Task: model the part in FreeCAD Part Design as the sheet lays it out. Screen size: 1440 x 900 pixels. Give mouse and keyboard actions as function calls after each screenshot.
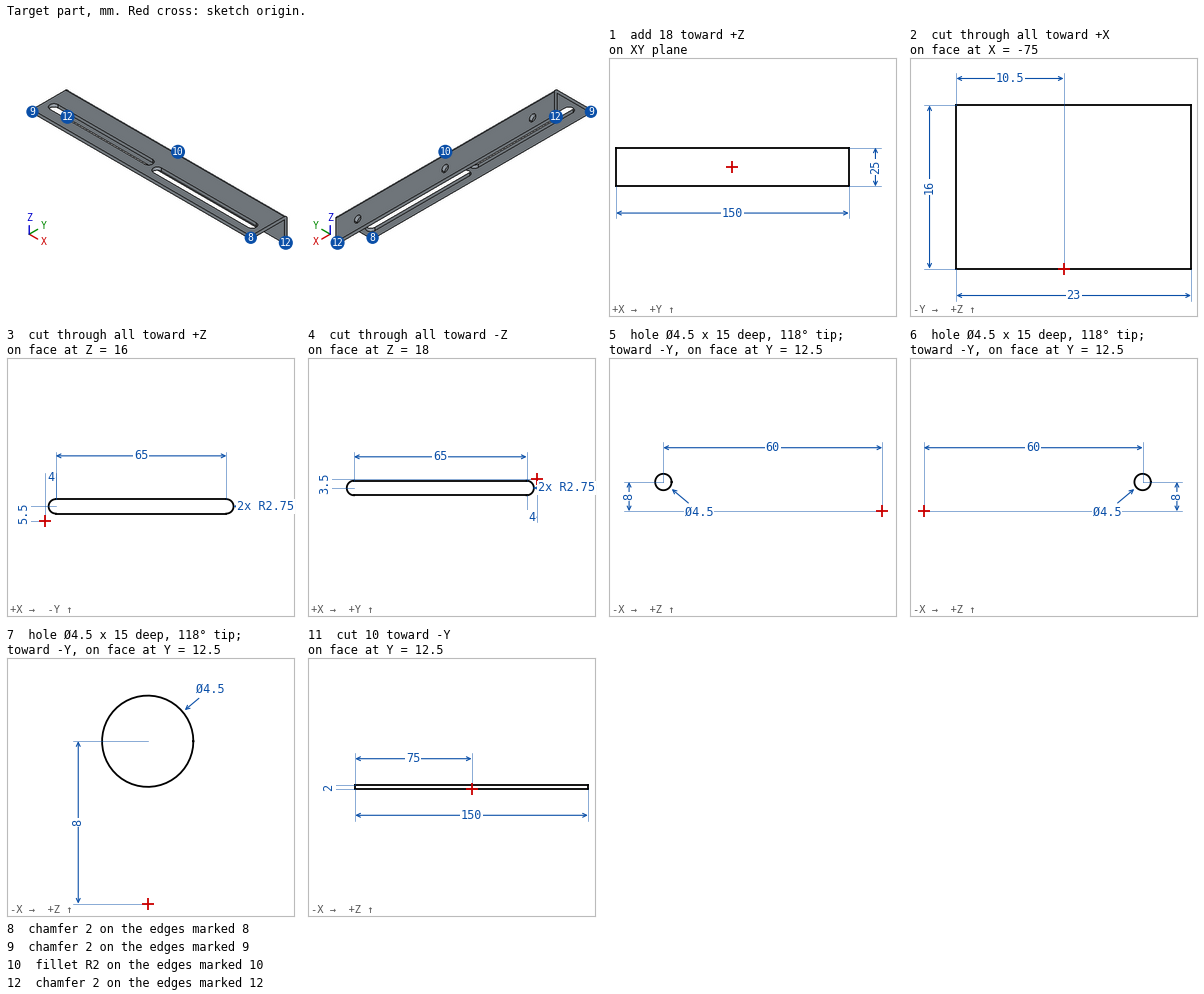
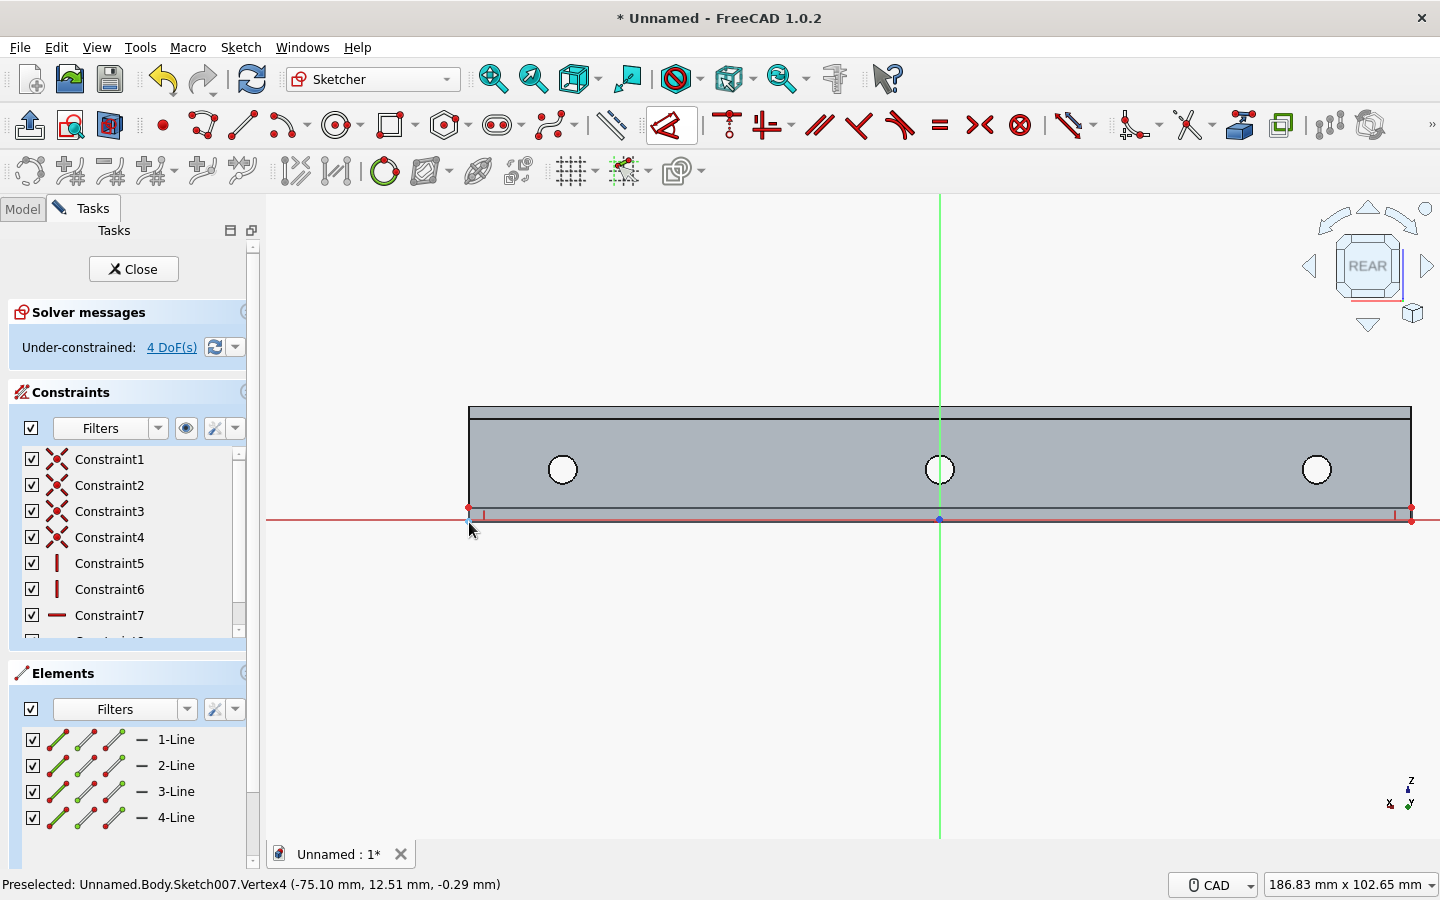
click(469, 522)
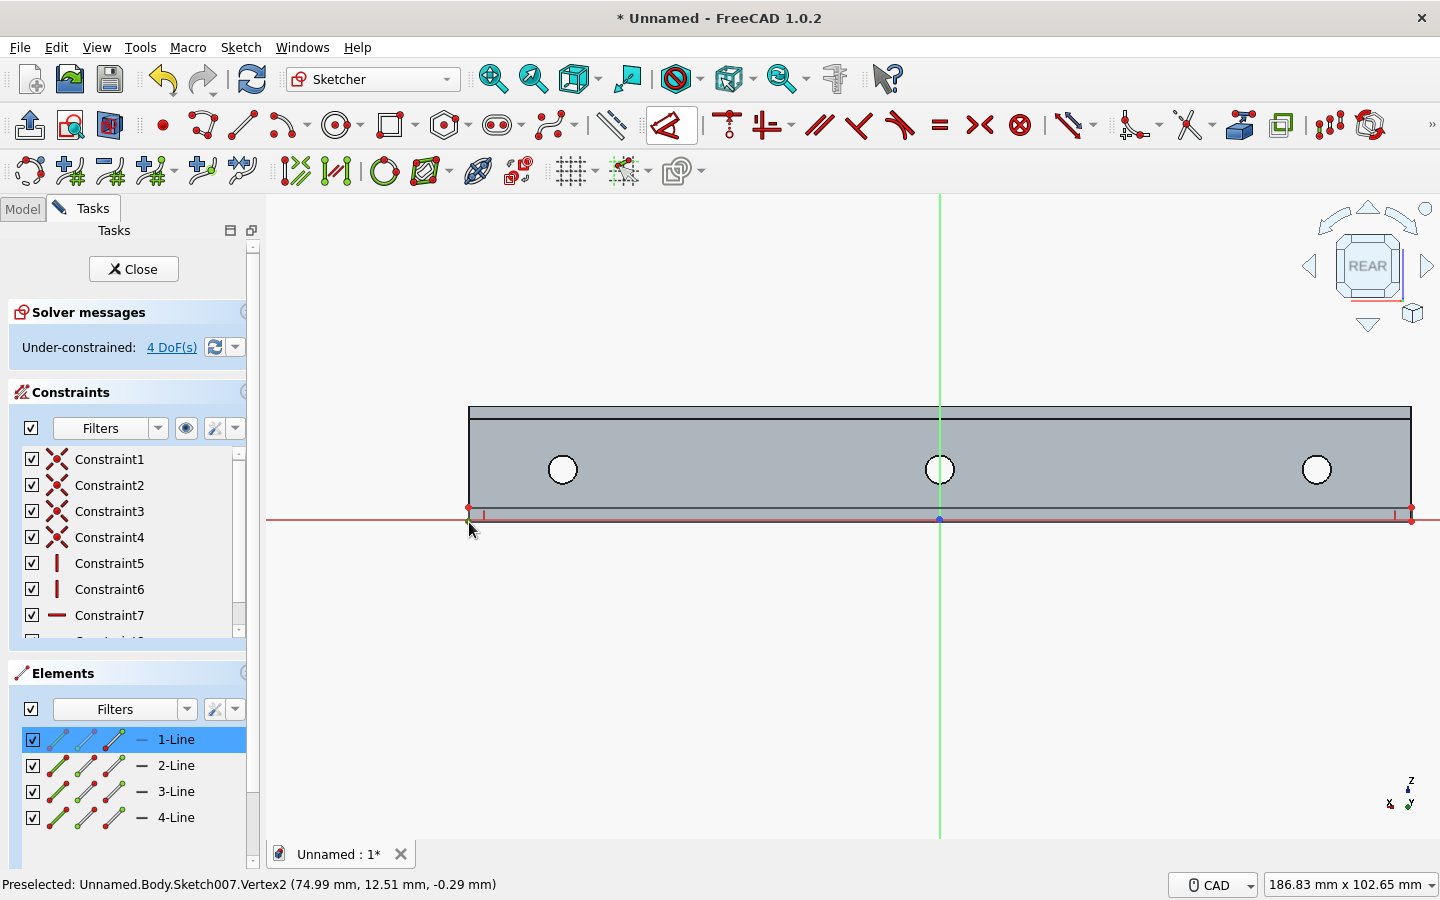
click(364, 520)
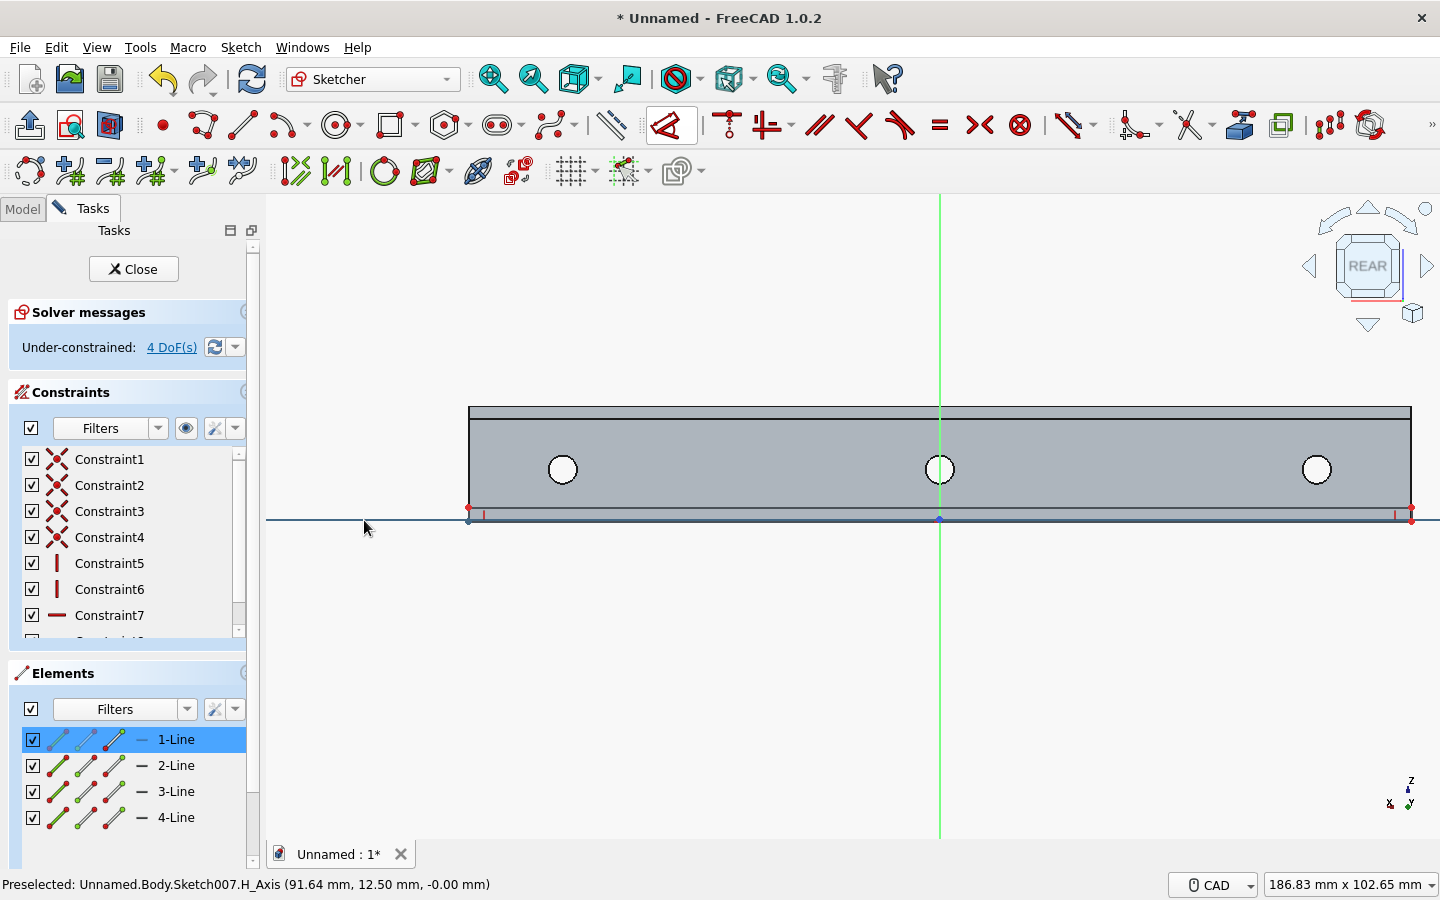
click(728, 126)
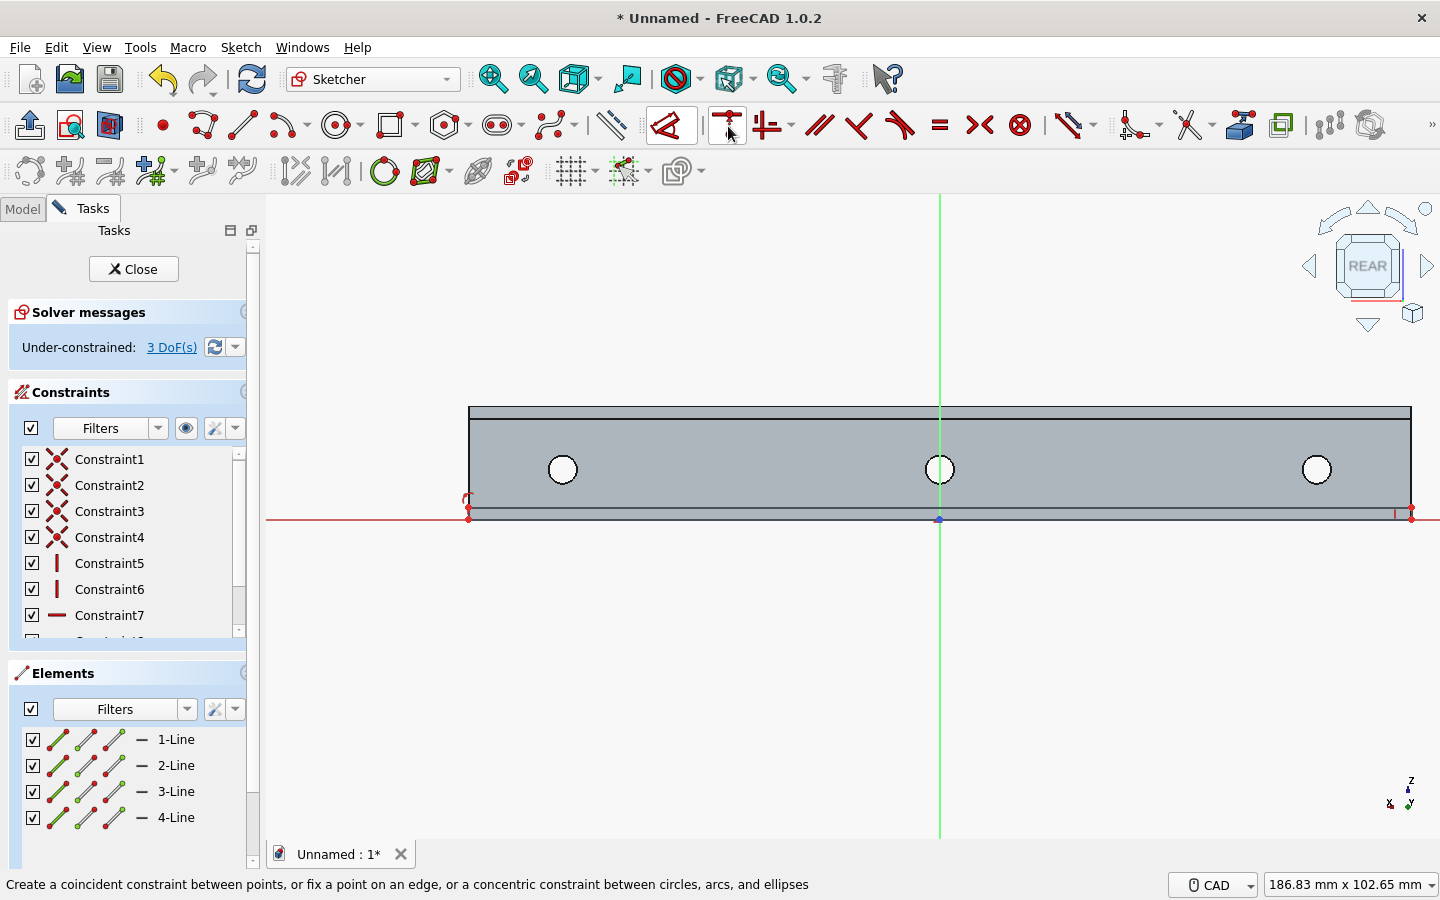
scroll(469, 514, up, 6)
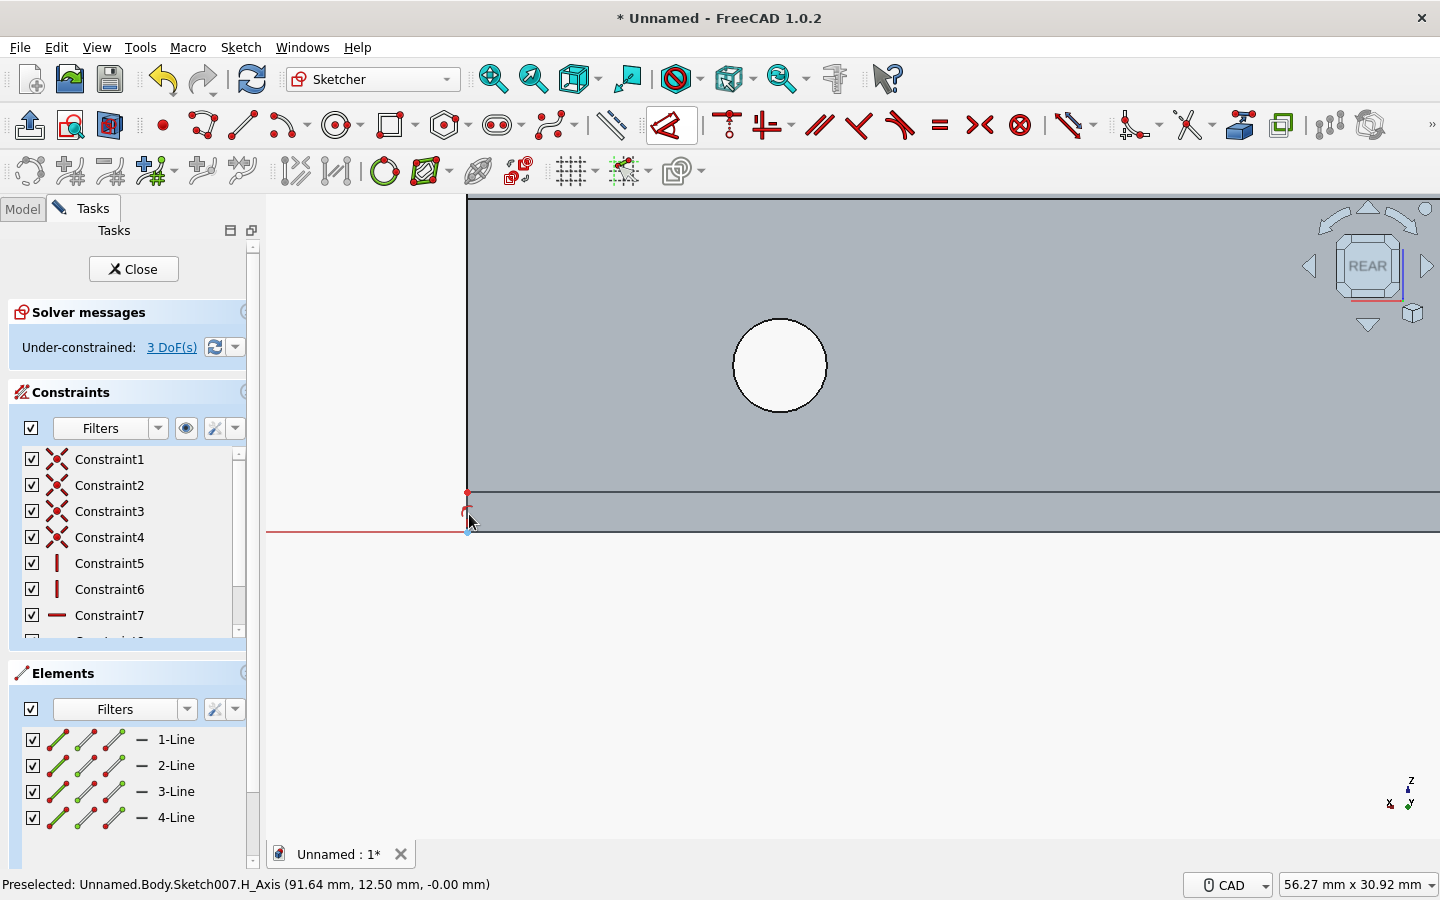
click(467, 500)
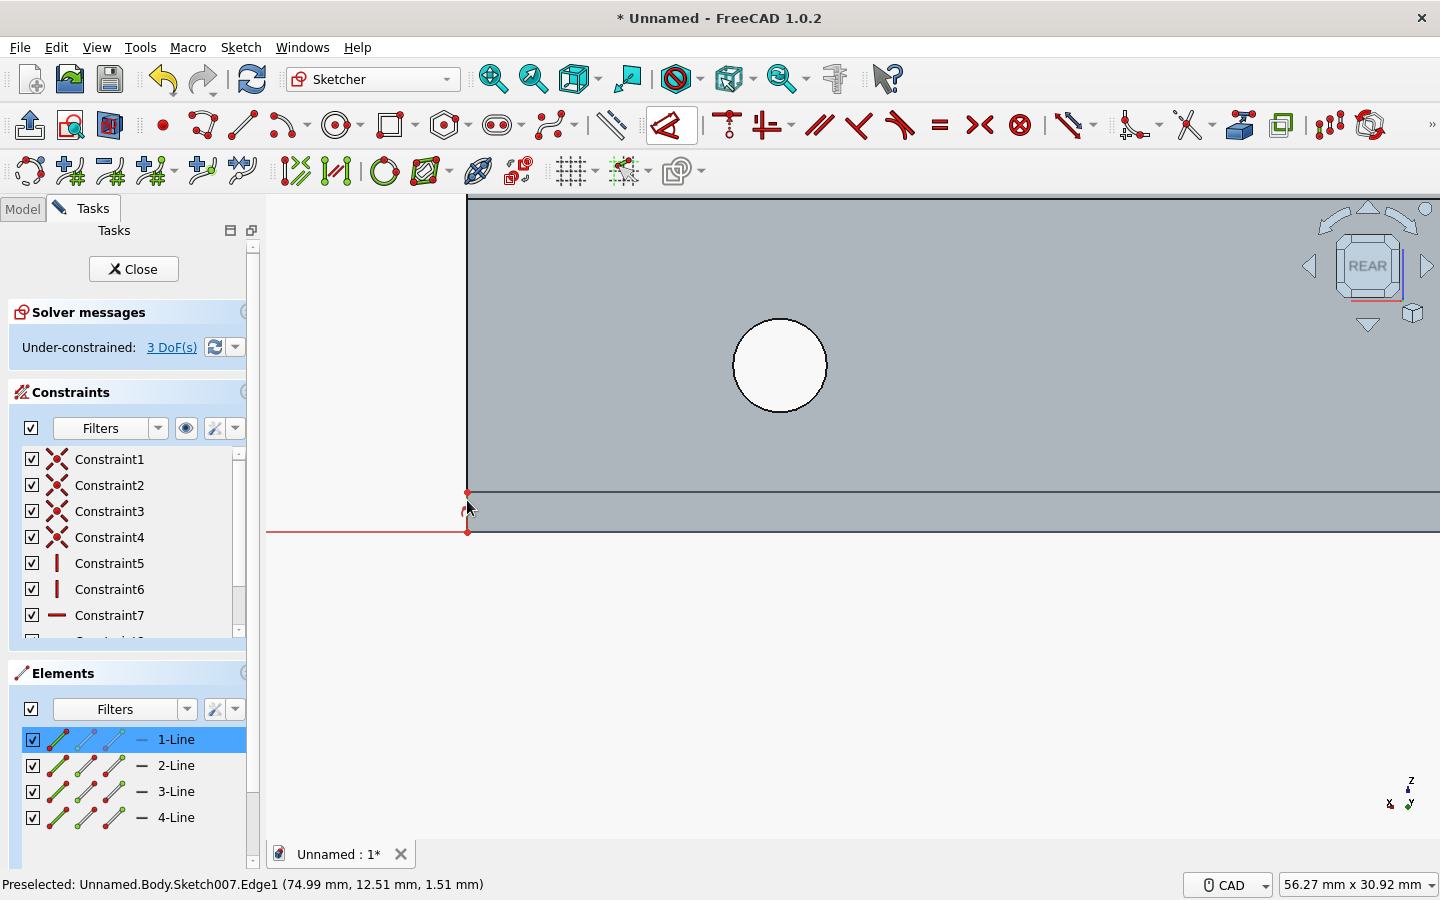
key(i)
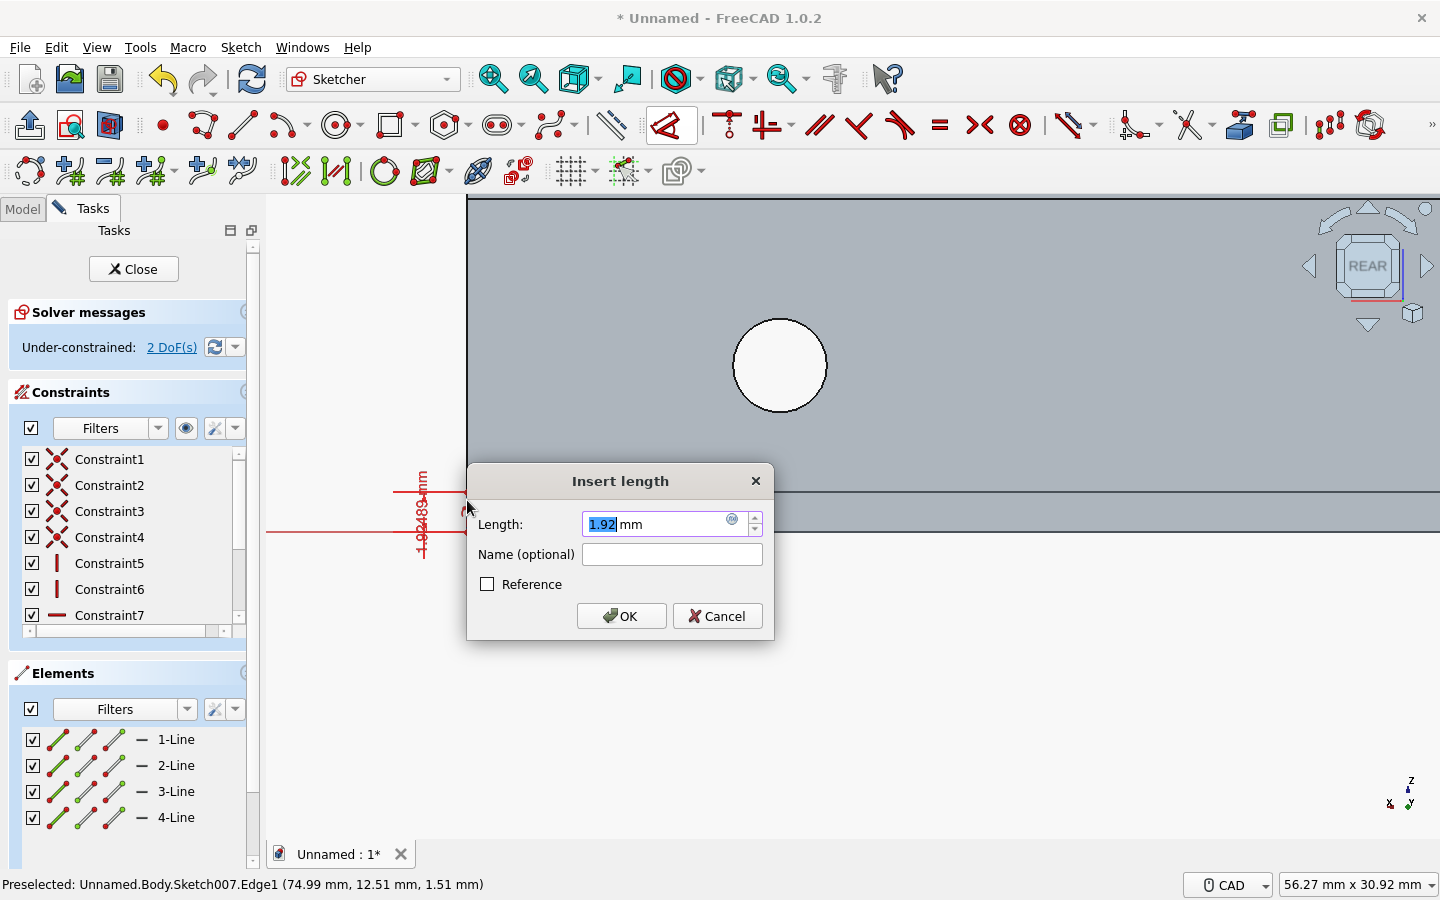
text(2)
key(Return)